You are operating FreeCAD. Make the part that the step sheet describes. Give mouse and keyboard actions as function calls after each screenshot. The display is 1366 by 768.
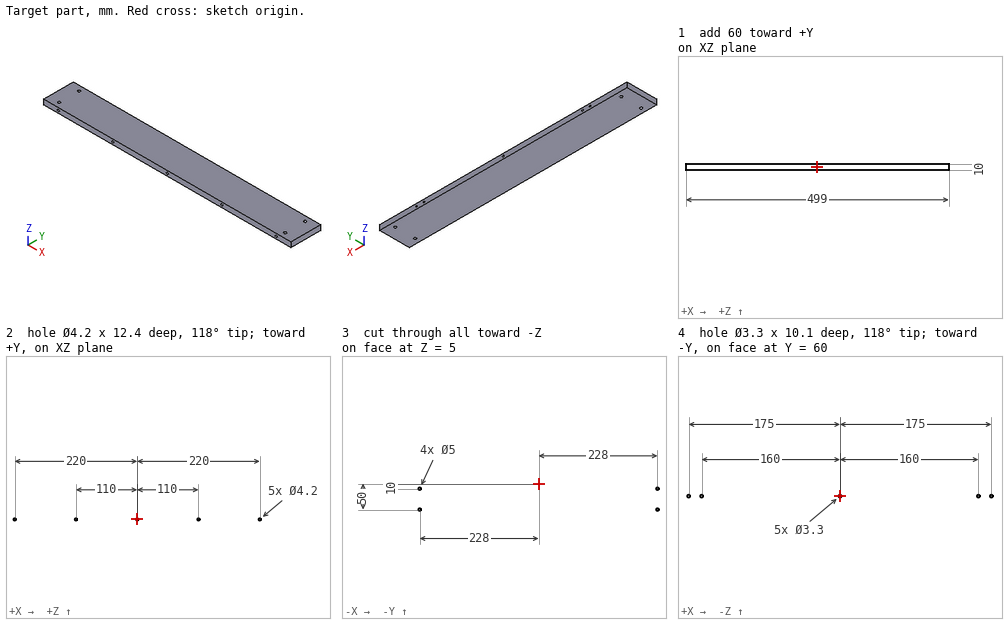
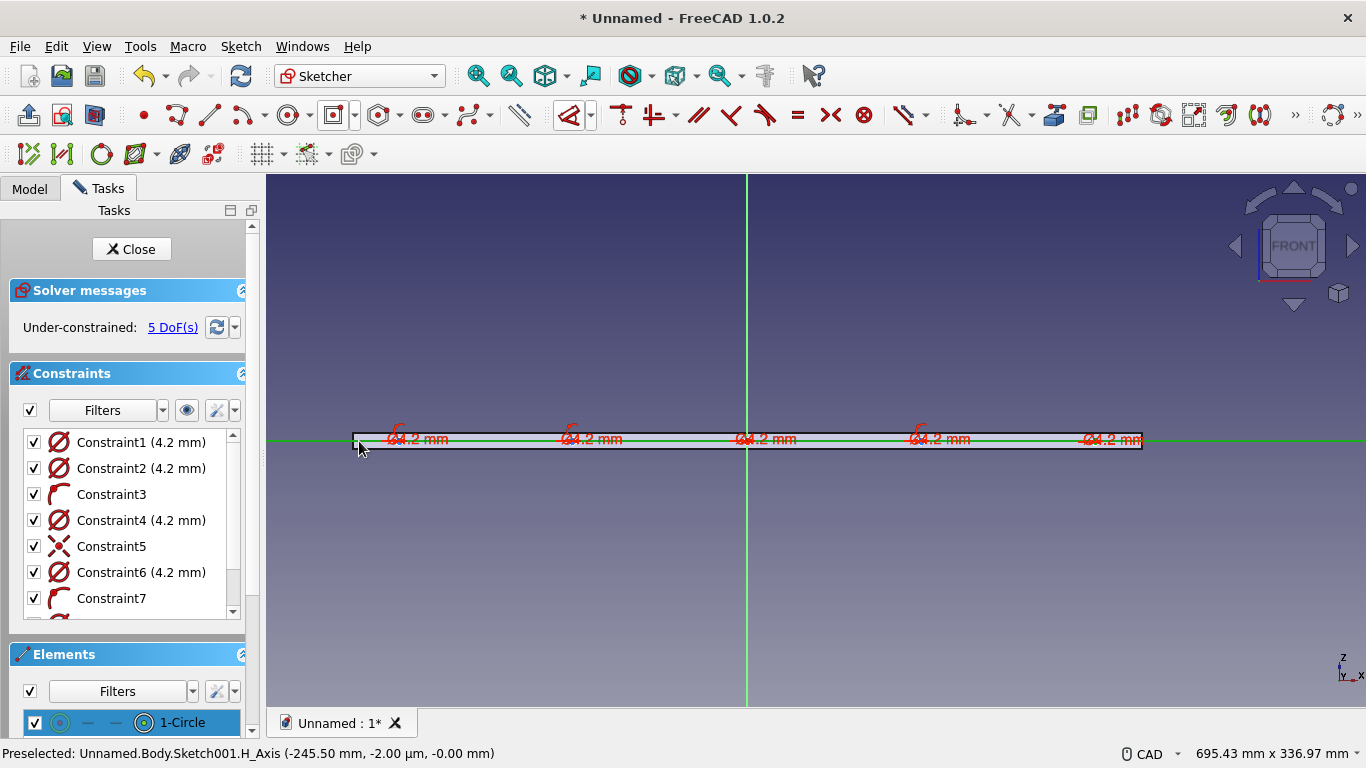
key(c)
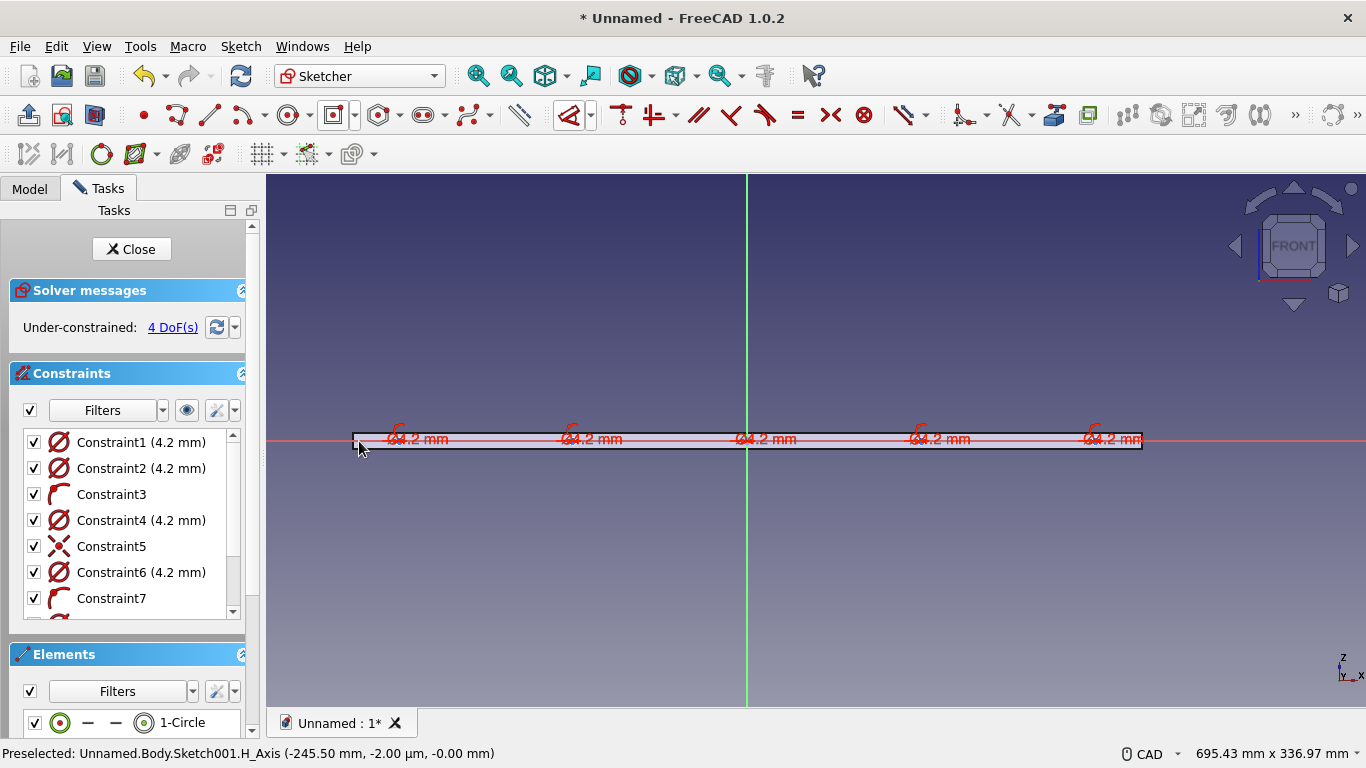
click(568, 116)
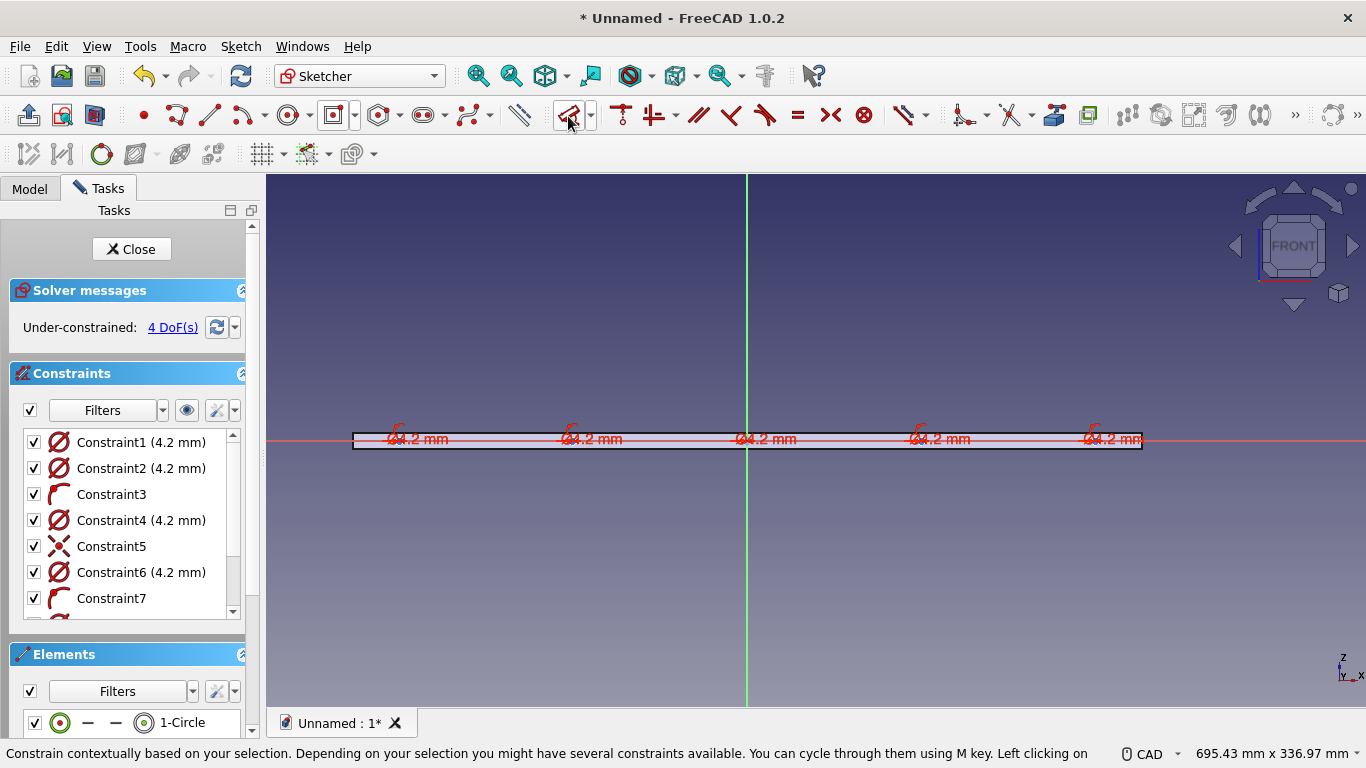
click(1095, 441)
click(921, 475)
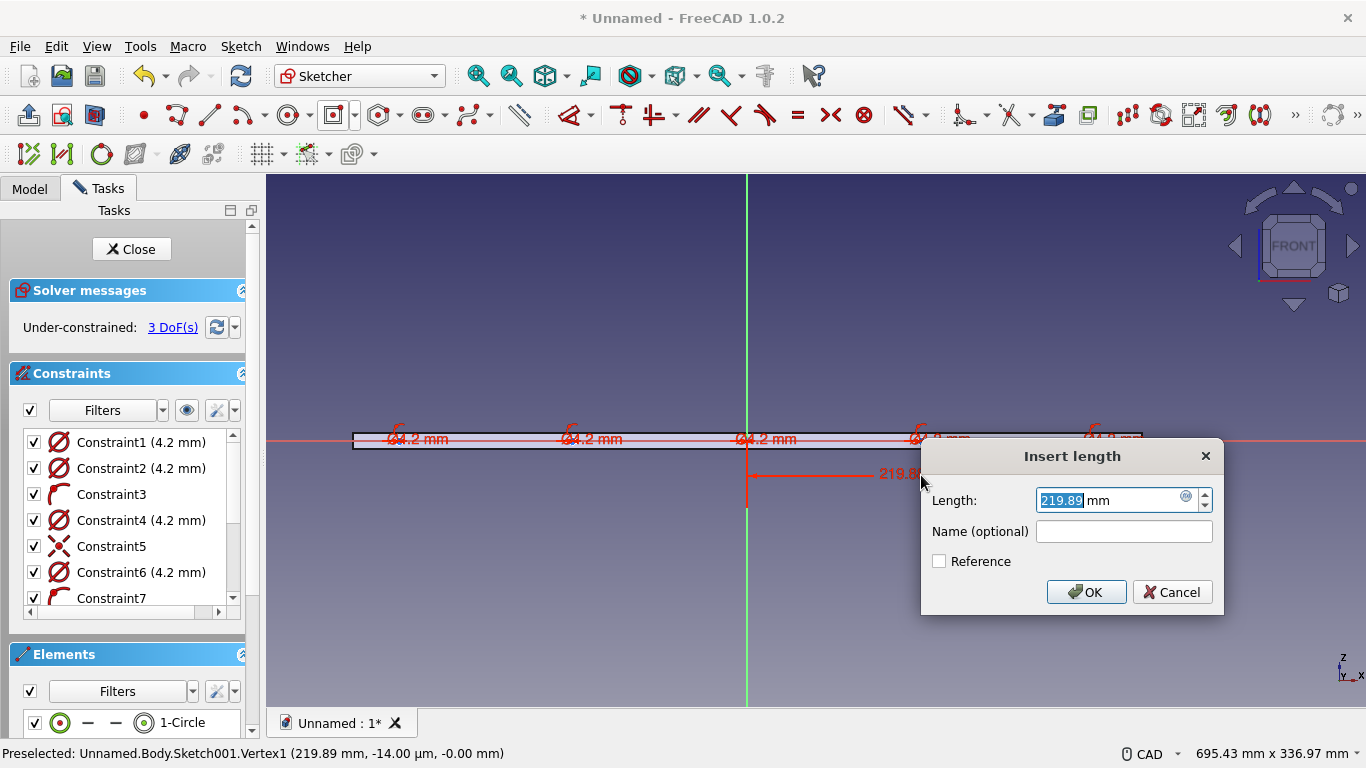
text(220)
key(Return)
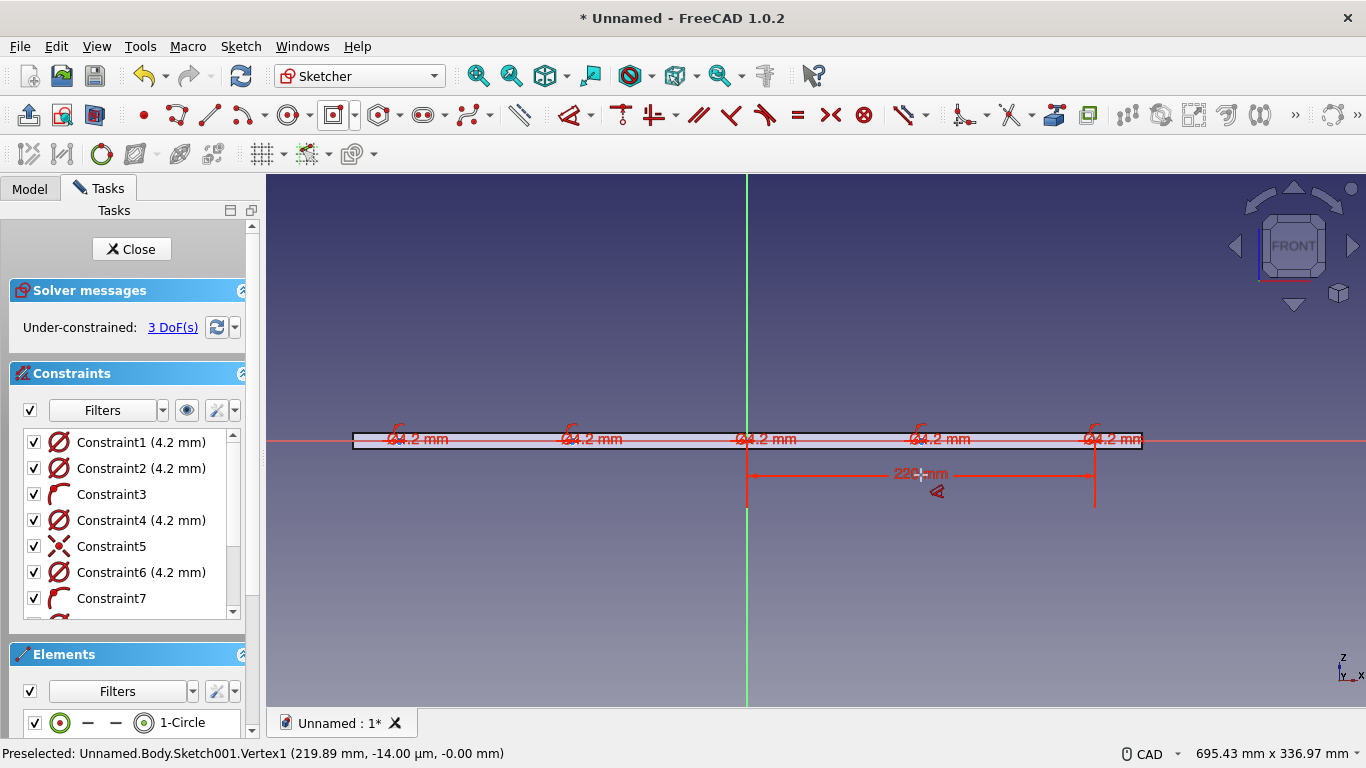
click(921, 441)
click(834, 475)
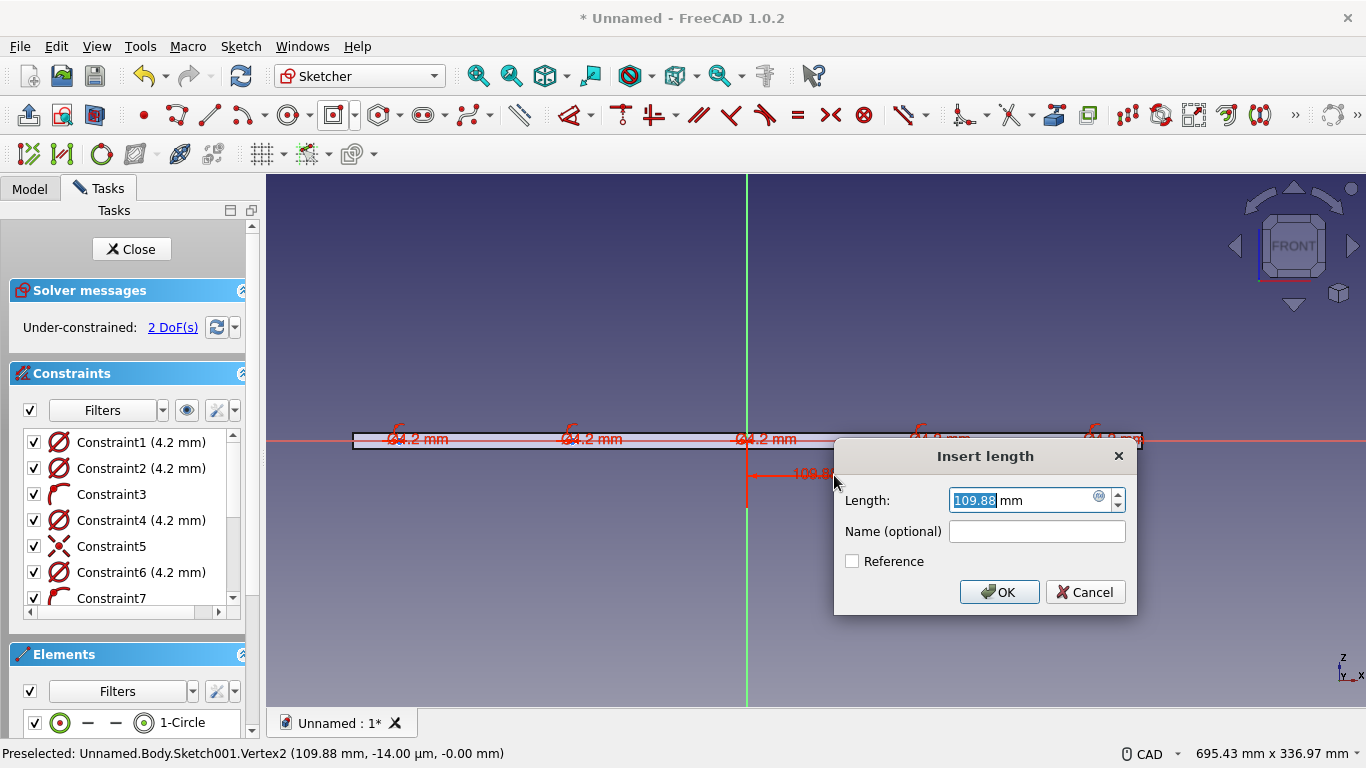
text(110)
key(Return)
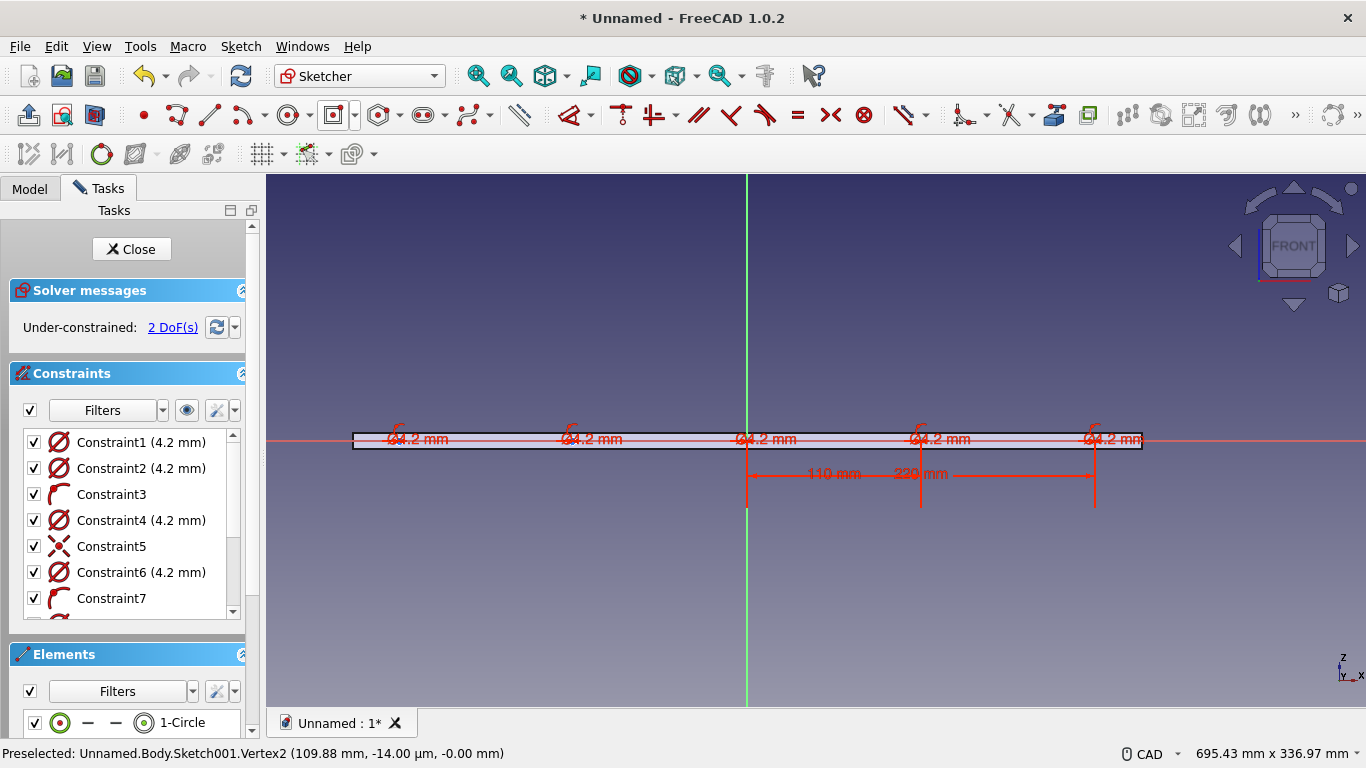
click(573, 441)
click(660, 475)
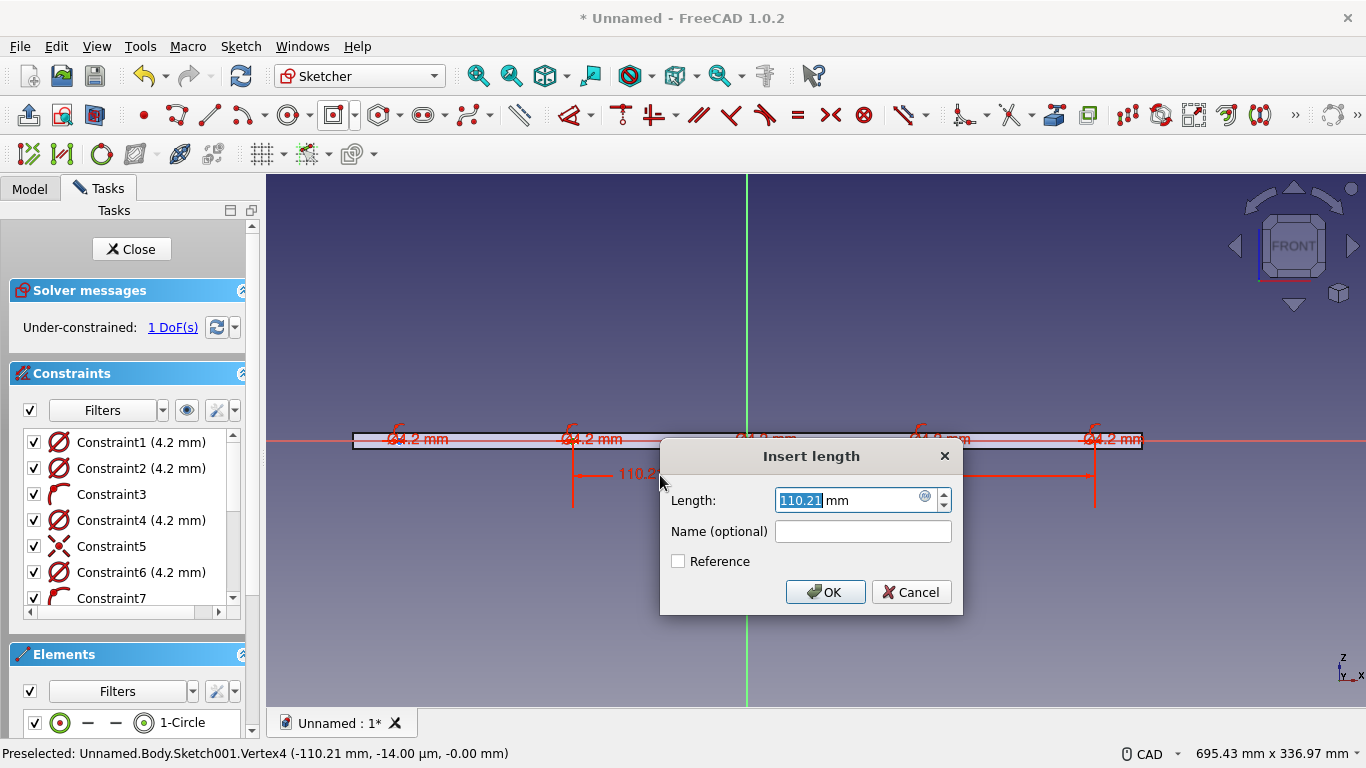
text(110)
key(Return)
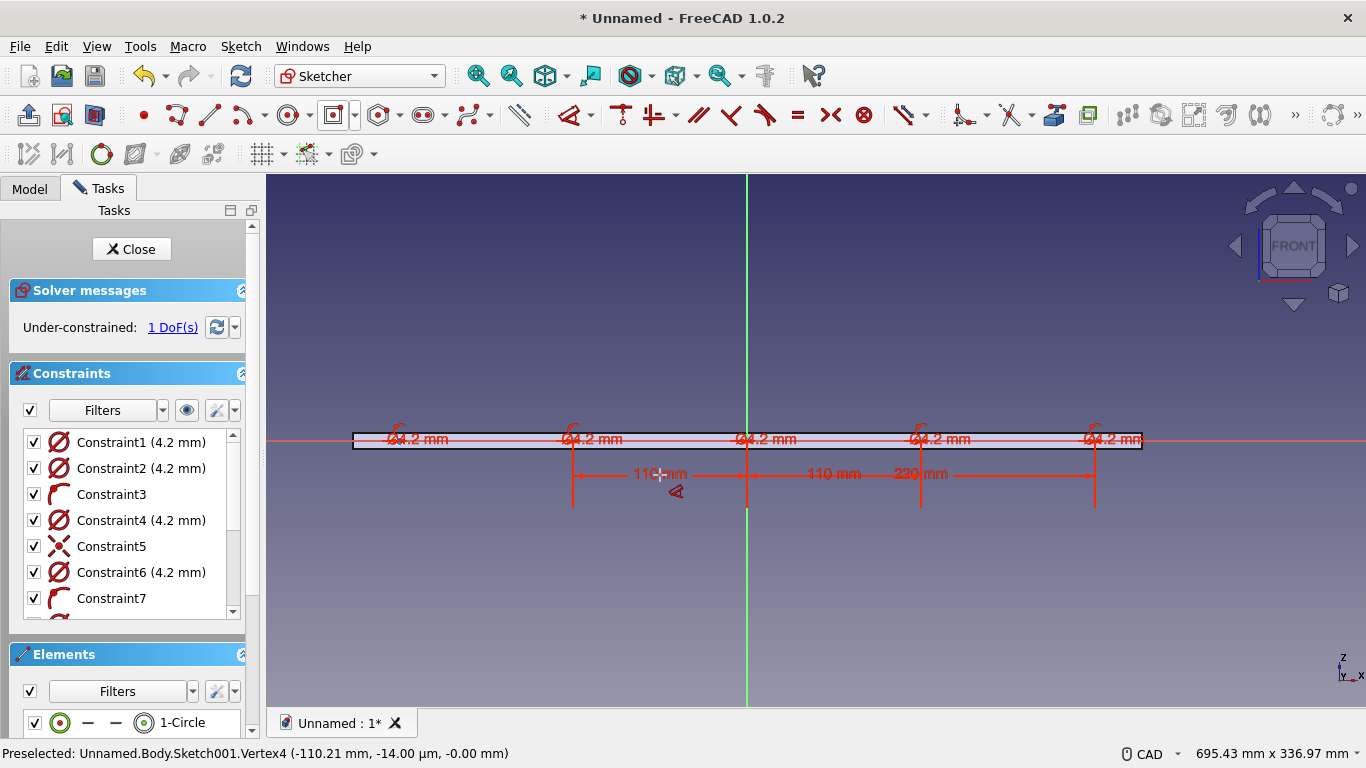
click(399, 441)
click(573, 475)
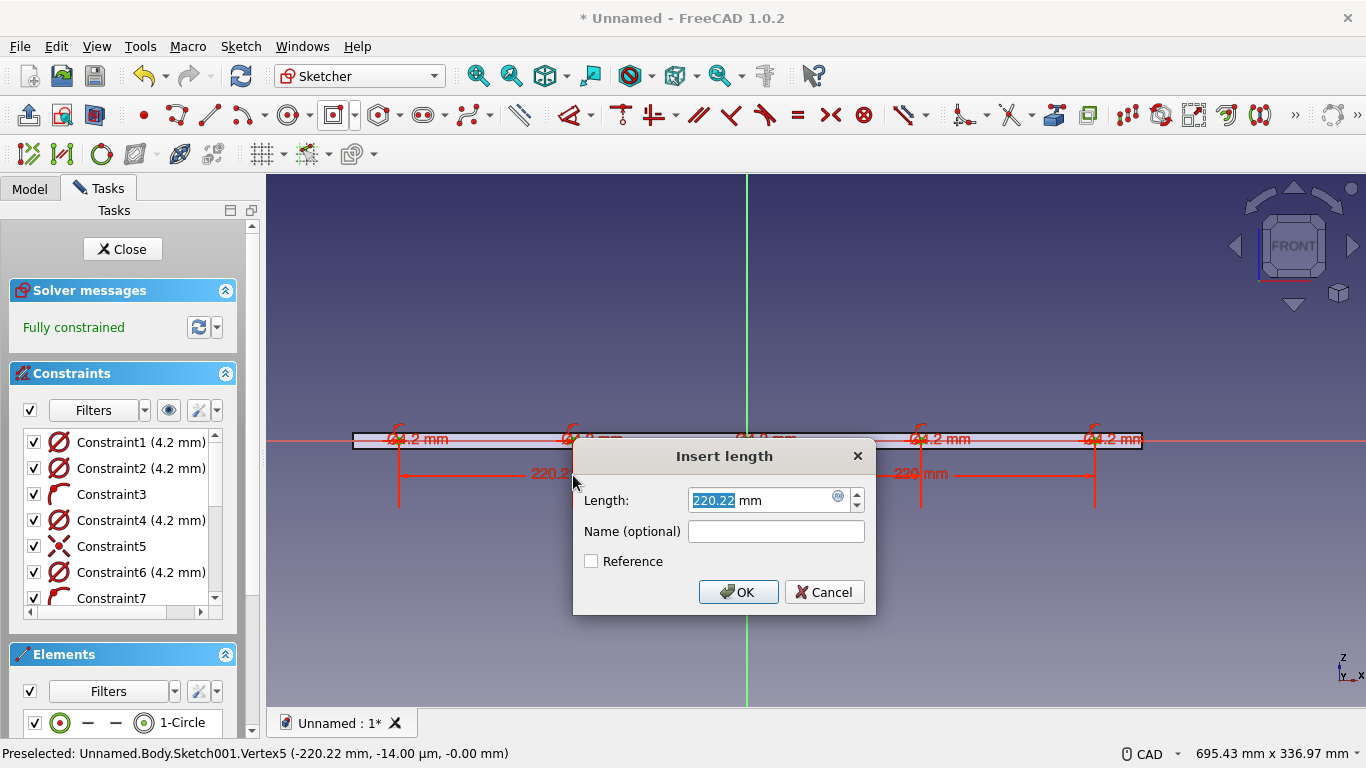
text(220)
key(Return)
key(Escape)